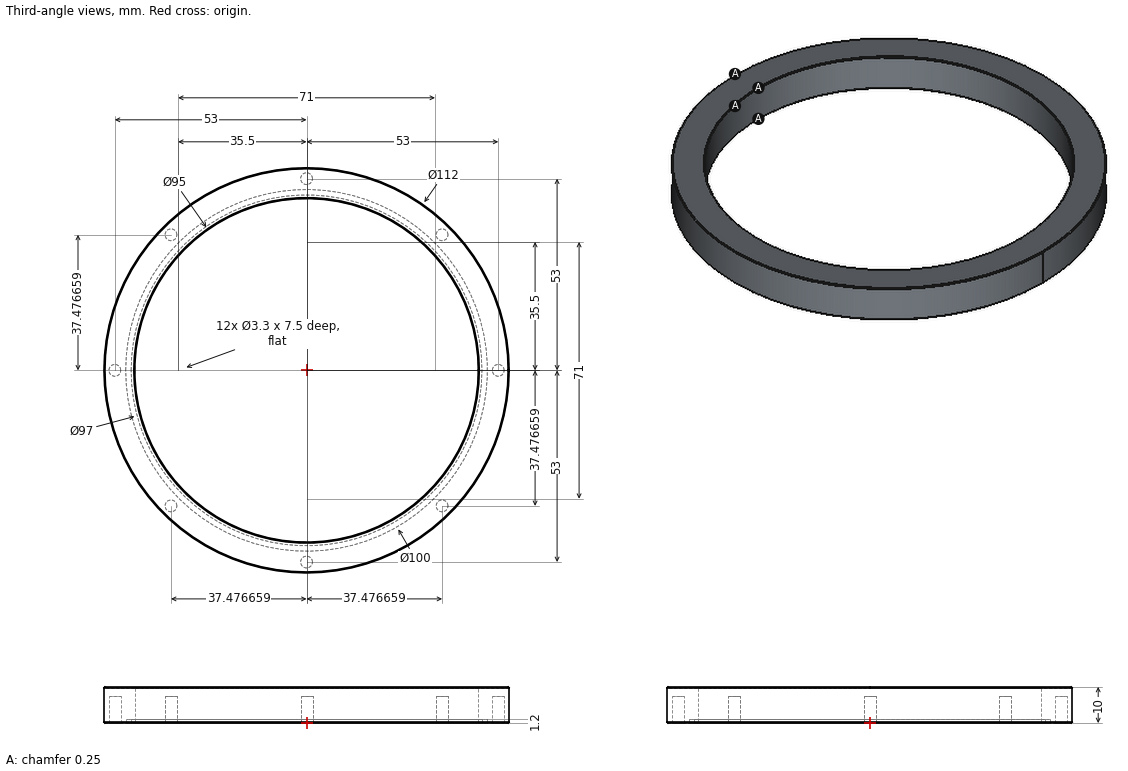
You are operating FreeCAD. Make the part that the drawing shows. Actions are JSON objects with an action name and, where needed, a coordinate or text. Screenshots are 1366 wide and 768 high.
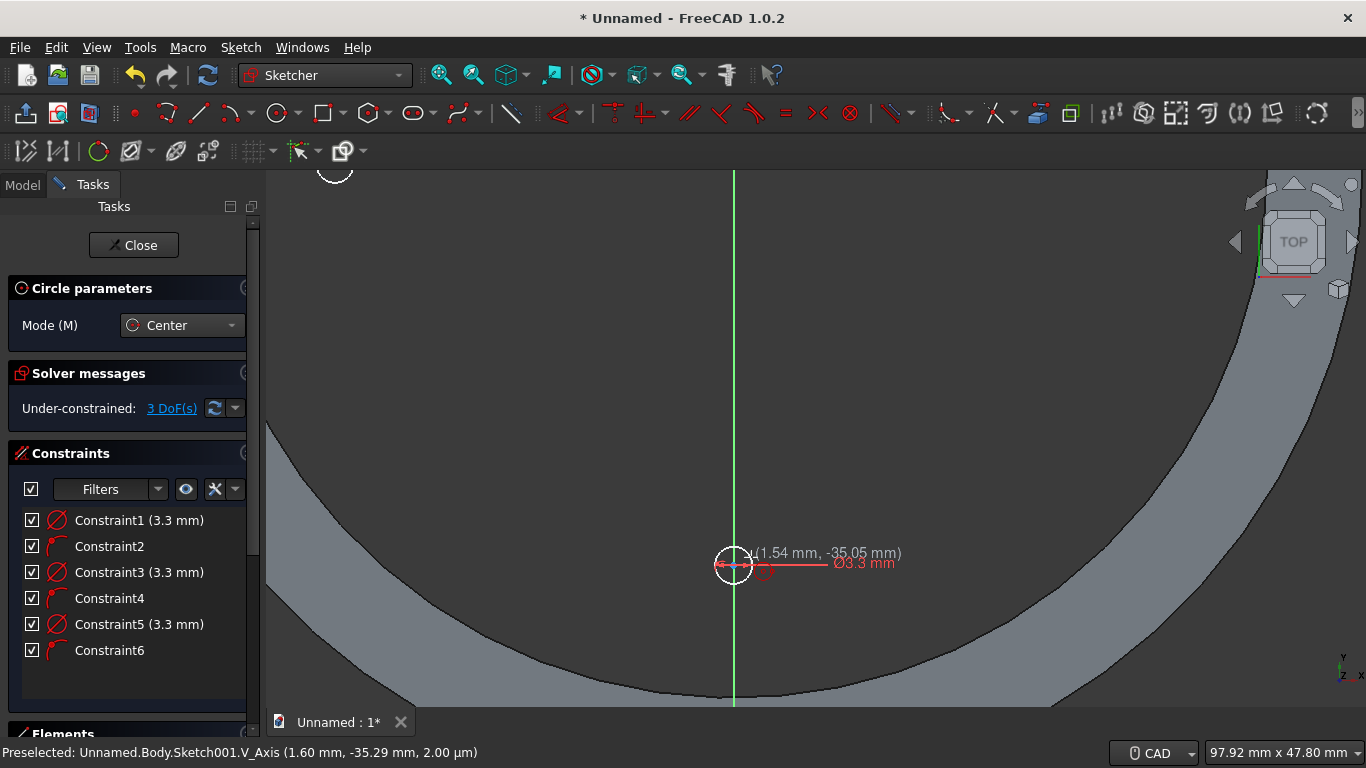
{"action": "scroll", "coordinate": [753, 557], "scroll_direction": "down", "scroll_amount": 6}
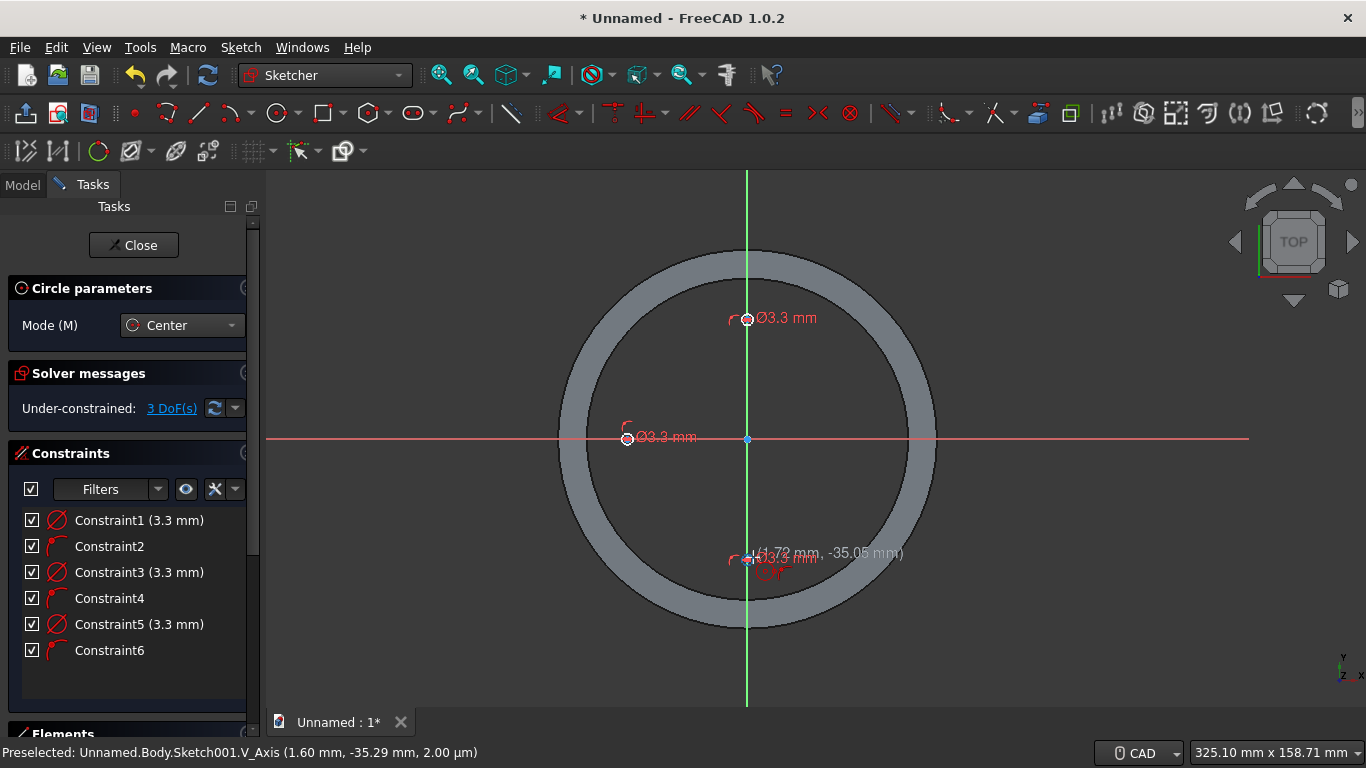
{"action": "scroll", "coordinate": [868, 439], "scroll_direction": "up", "scroll_amount": 8}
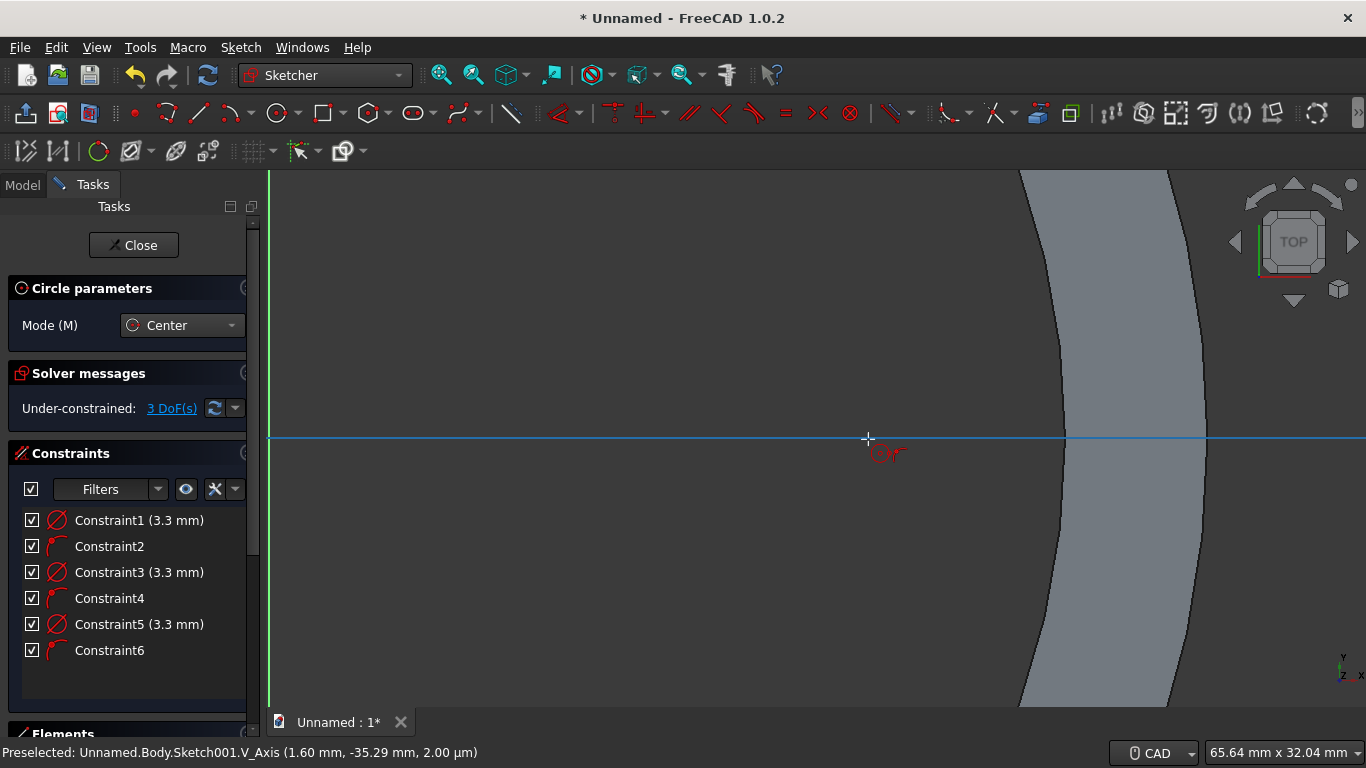
{"action": "scroll", "coordinate": [869, 439], "scroll_direction": "down", "scroll_amount": 8}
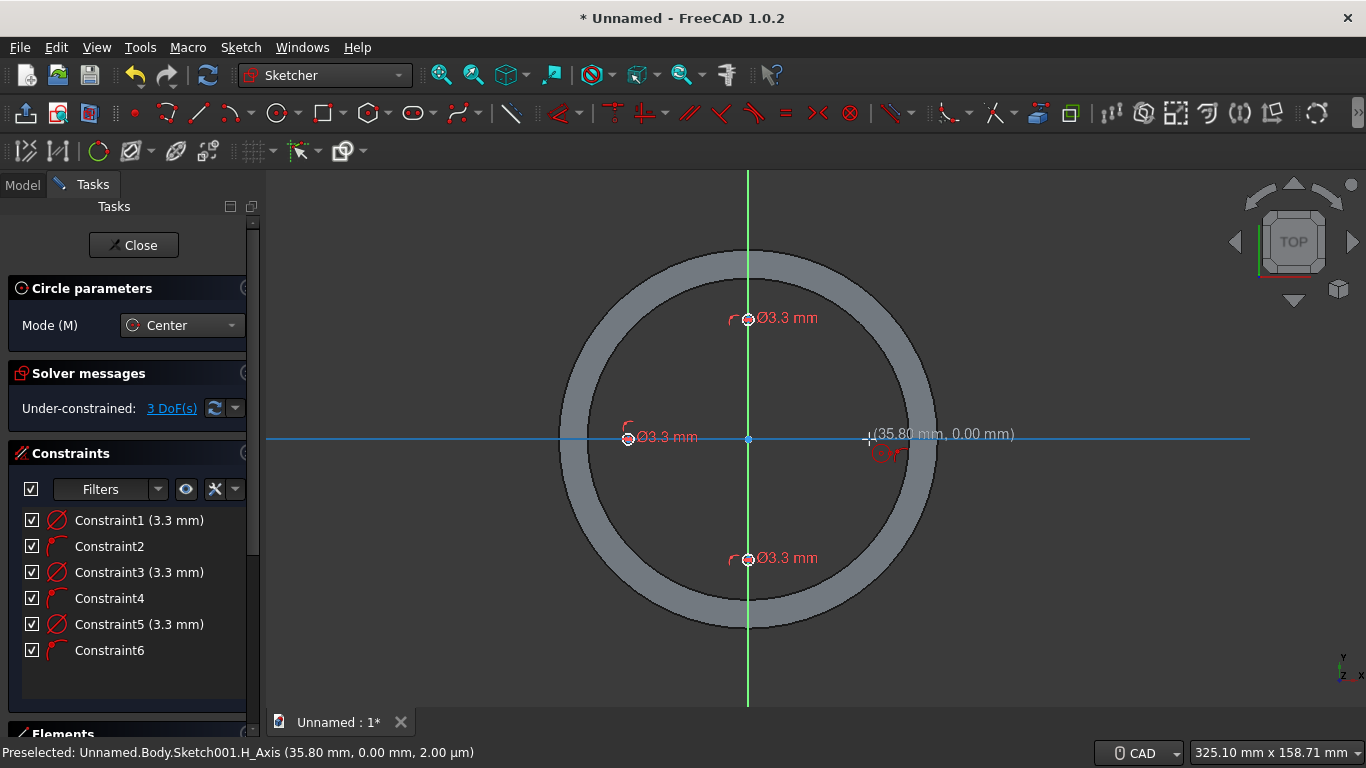
{"action": "left_click", "coordinate": [868, 439]}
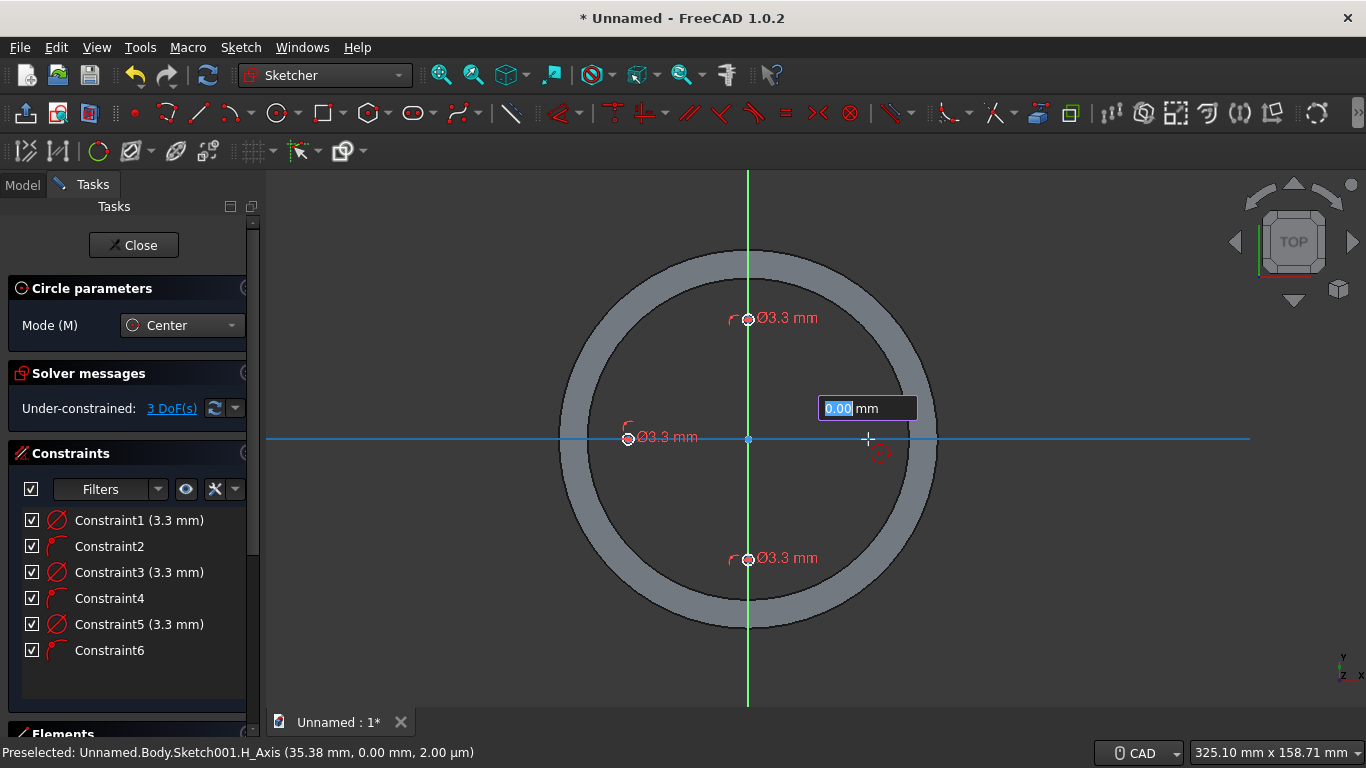
{"action": "scroll", "coordinate": [867, 444], "scroll_direction": "up", "scroll_amount": 6}
{"action": "mouse_move", "coordinate": [864, 444]}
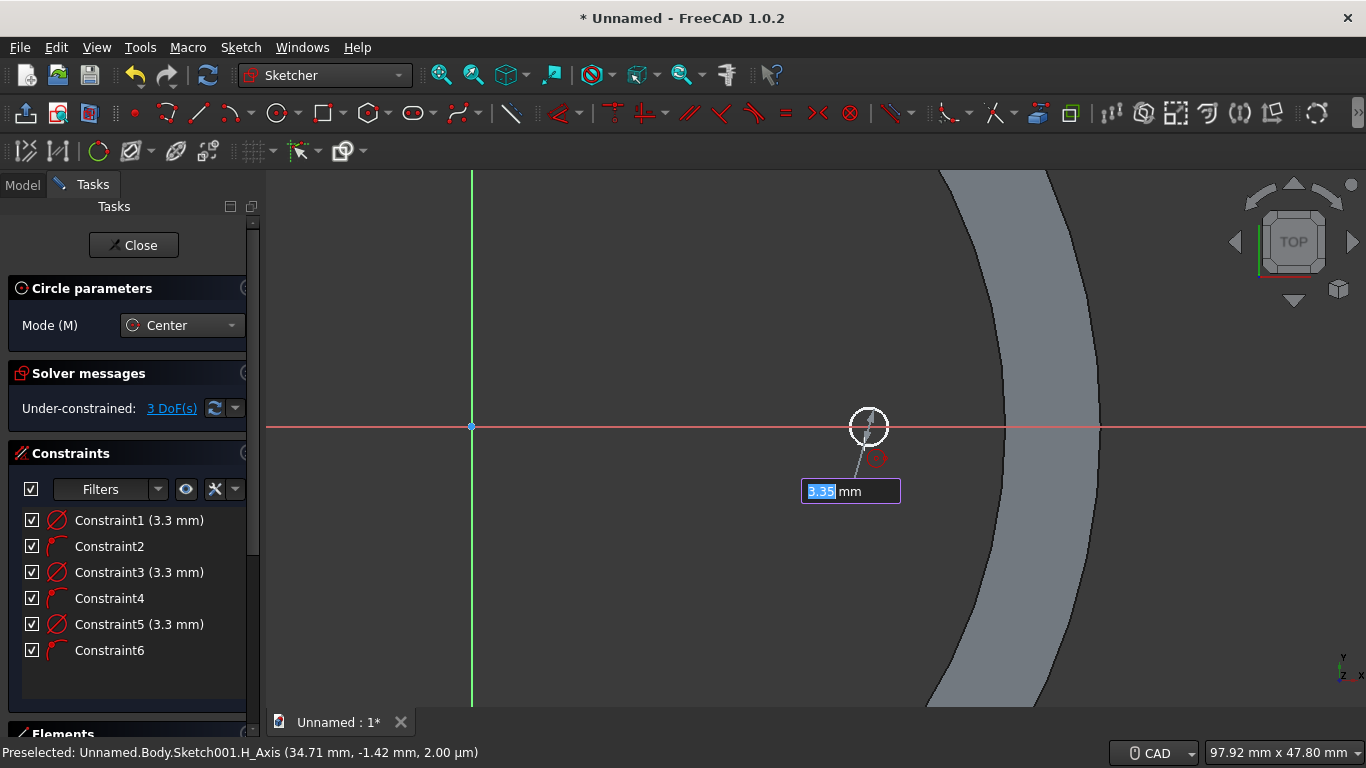
{"action": "type", "text": "3.3"}
{"action": "key", "text": "Return"}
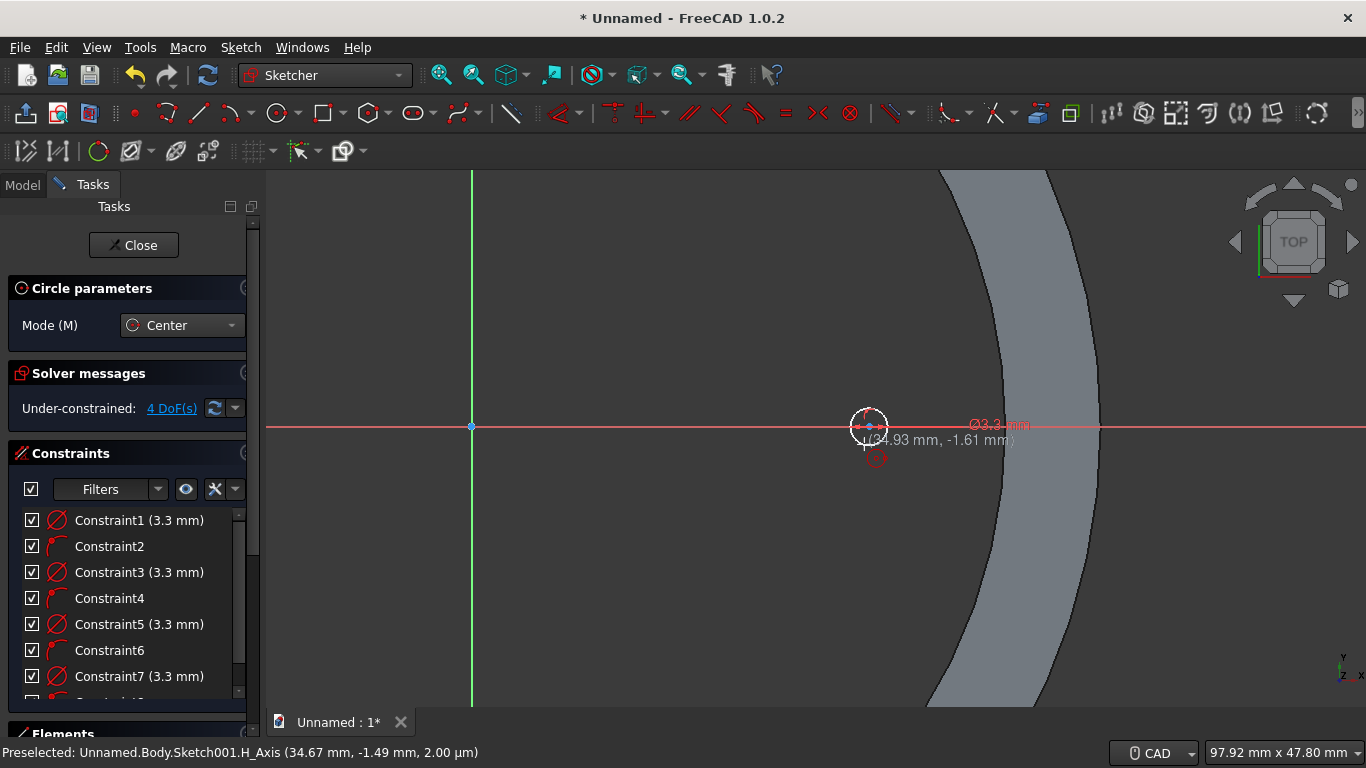
{"action": "scroll", "coordinate": [866, 444], "scroll_direction": "down", "scroll_amount": 6}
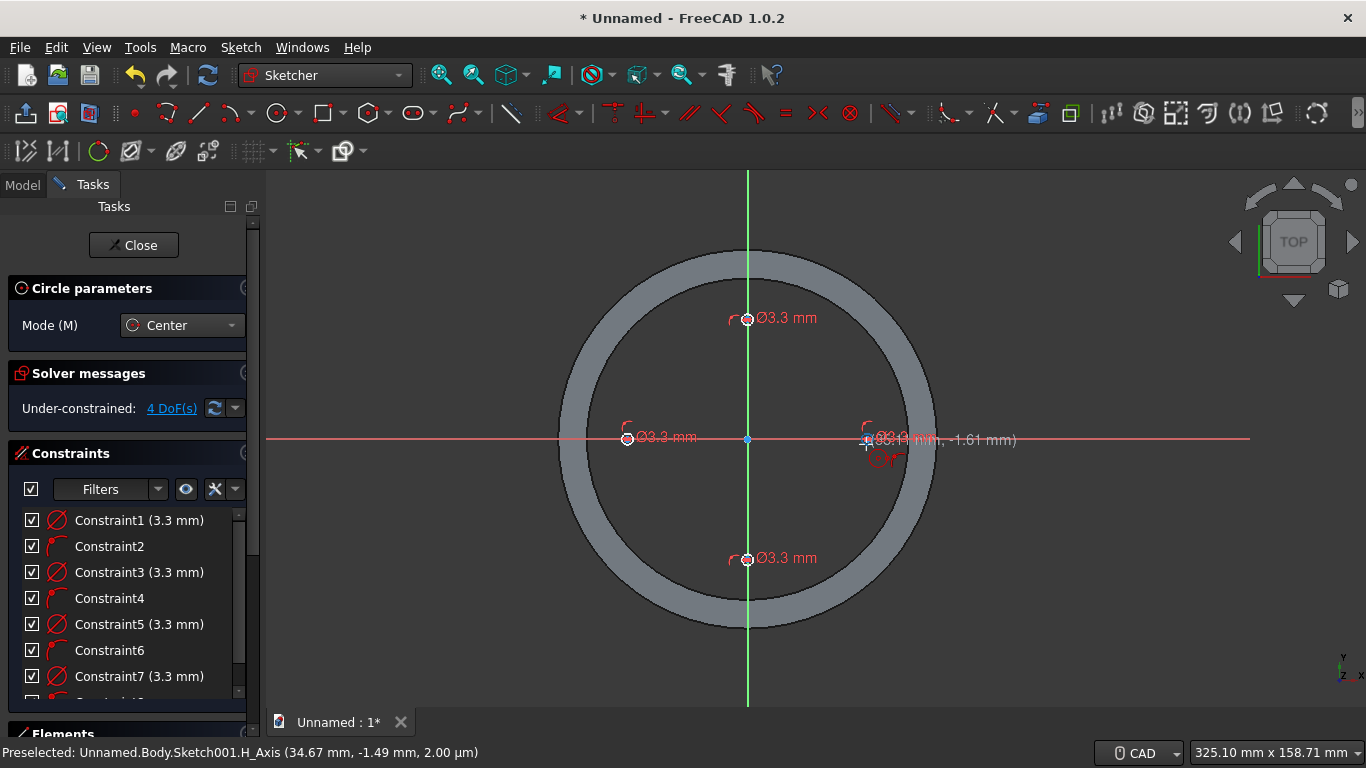
{"action": "scroll", "coordinate": [874, 566], "scroll_direction": "up", "scroll_amount": 8}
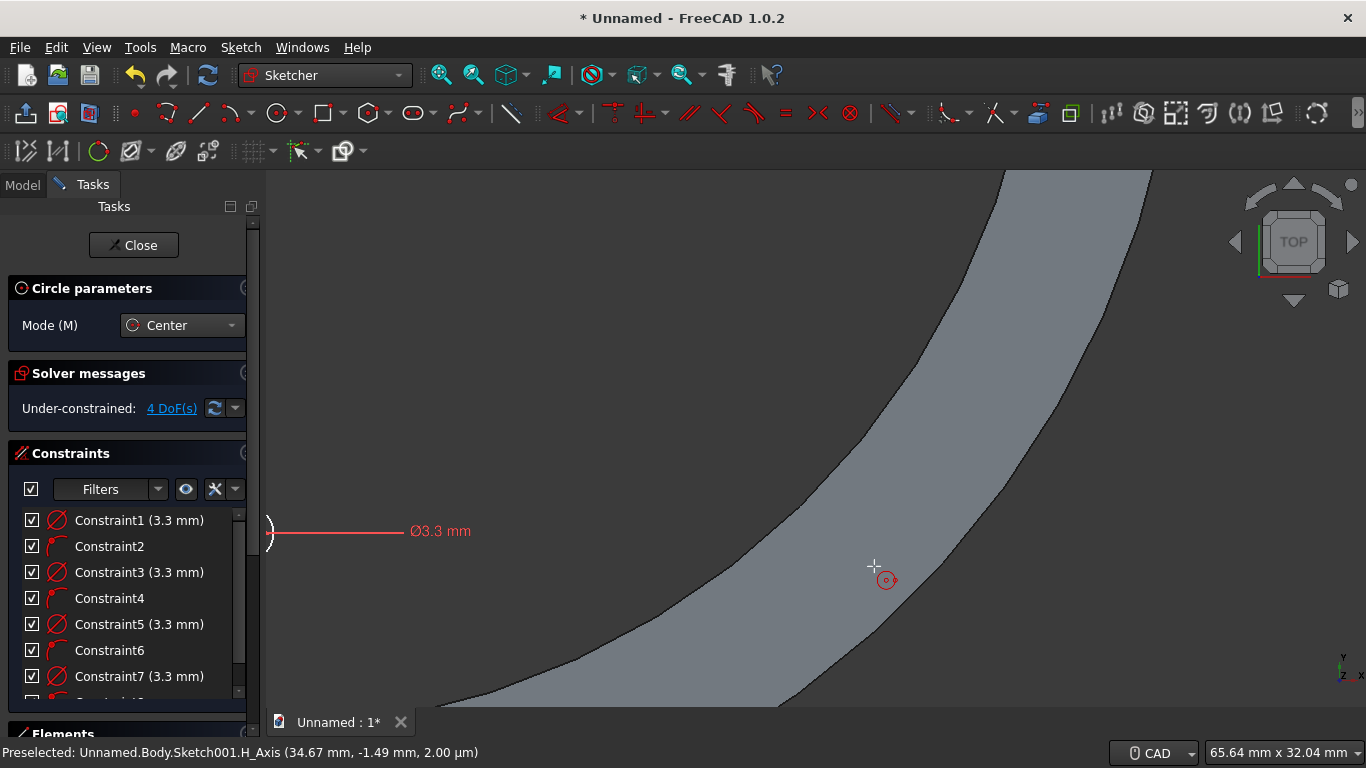
{"action": "scroll", "coordinate": [874, 566], "scroll_direction": "down", "scroll_amount": 8}